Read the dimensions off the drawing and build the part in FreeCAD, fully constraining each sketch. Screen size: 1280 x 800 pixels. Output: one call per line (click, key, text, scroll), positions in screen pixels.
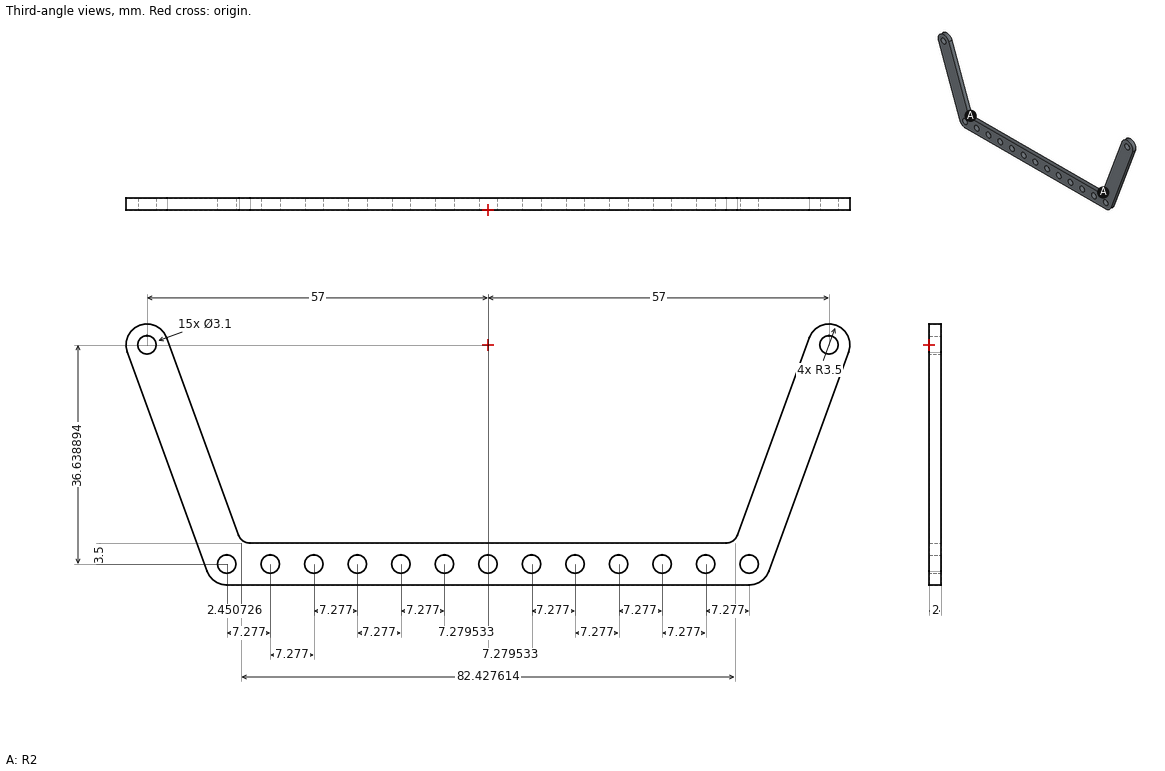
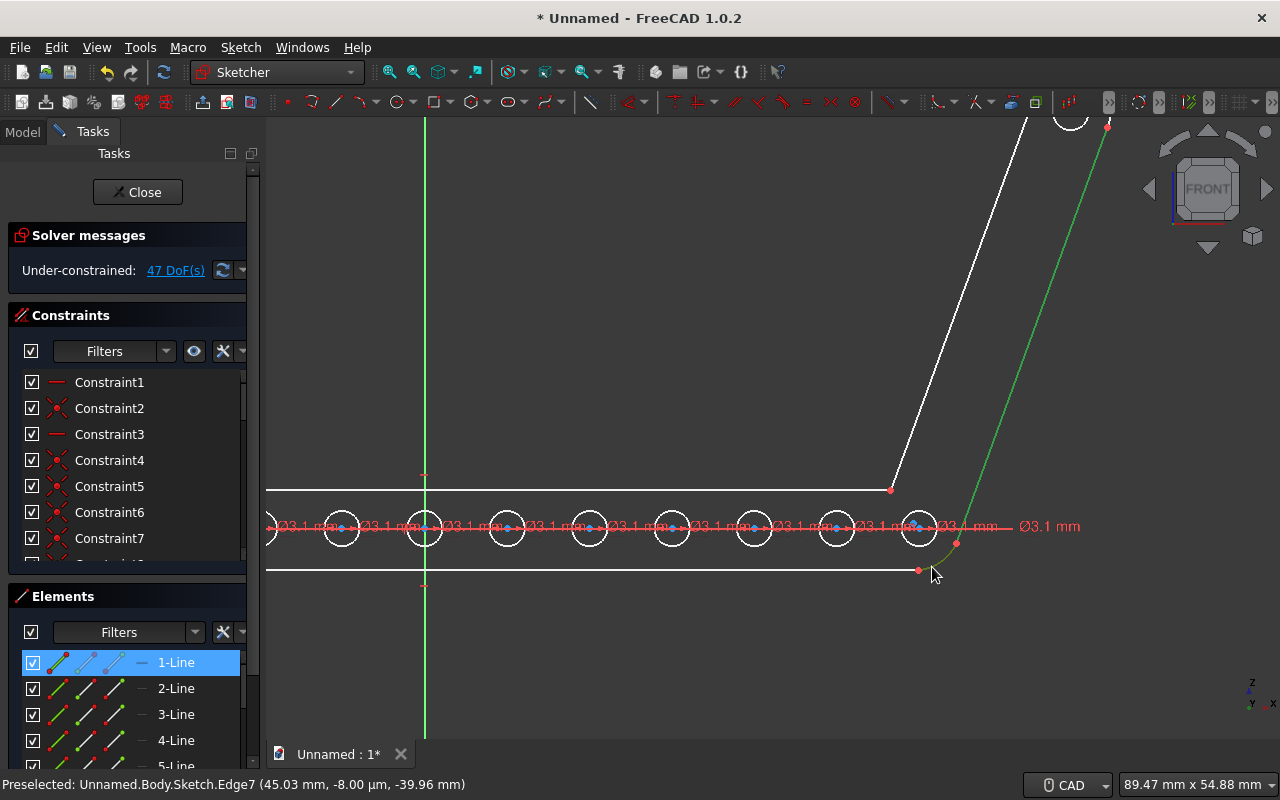
click(784, 102)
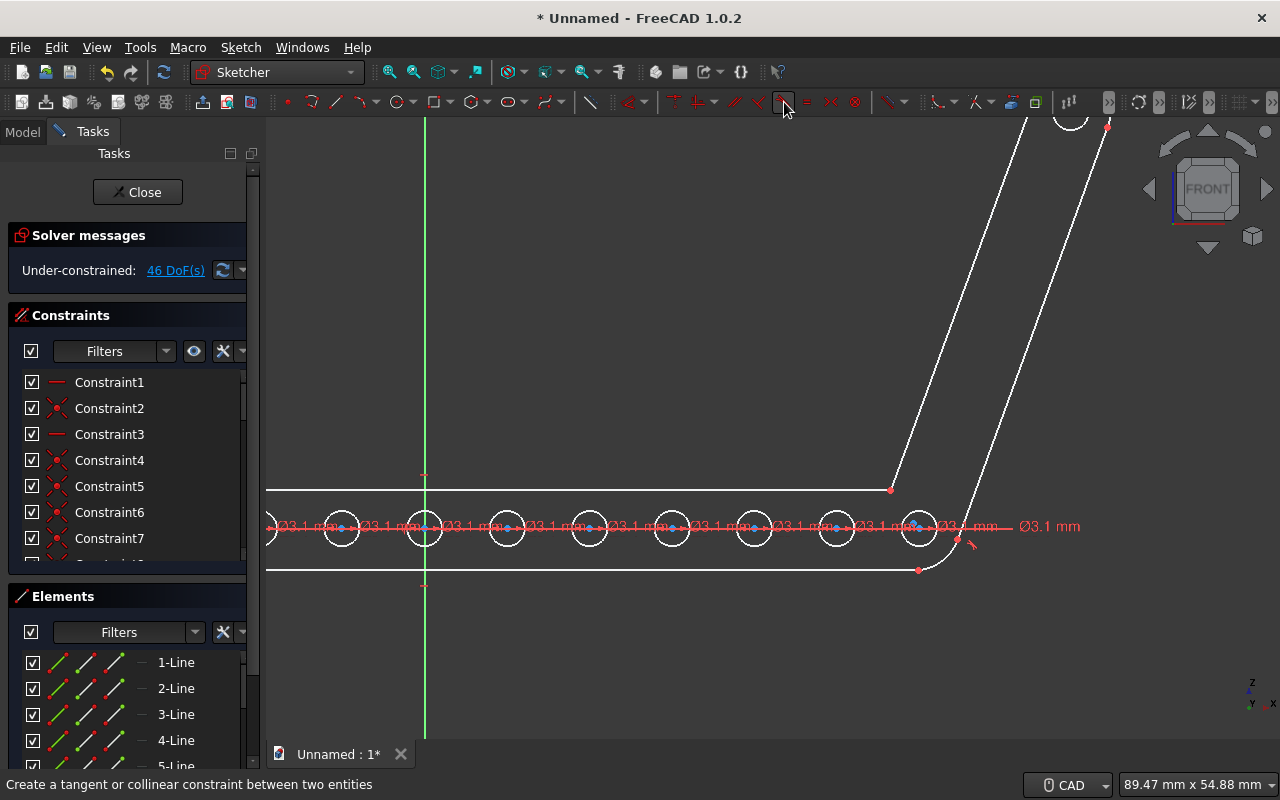
click(1063, 251)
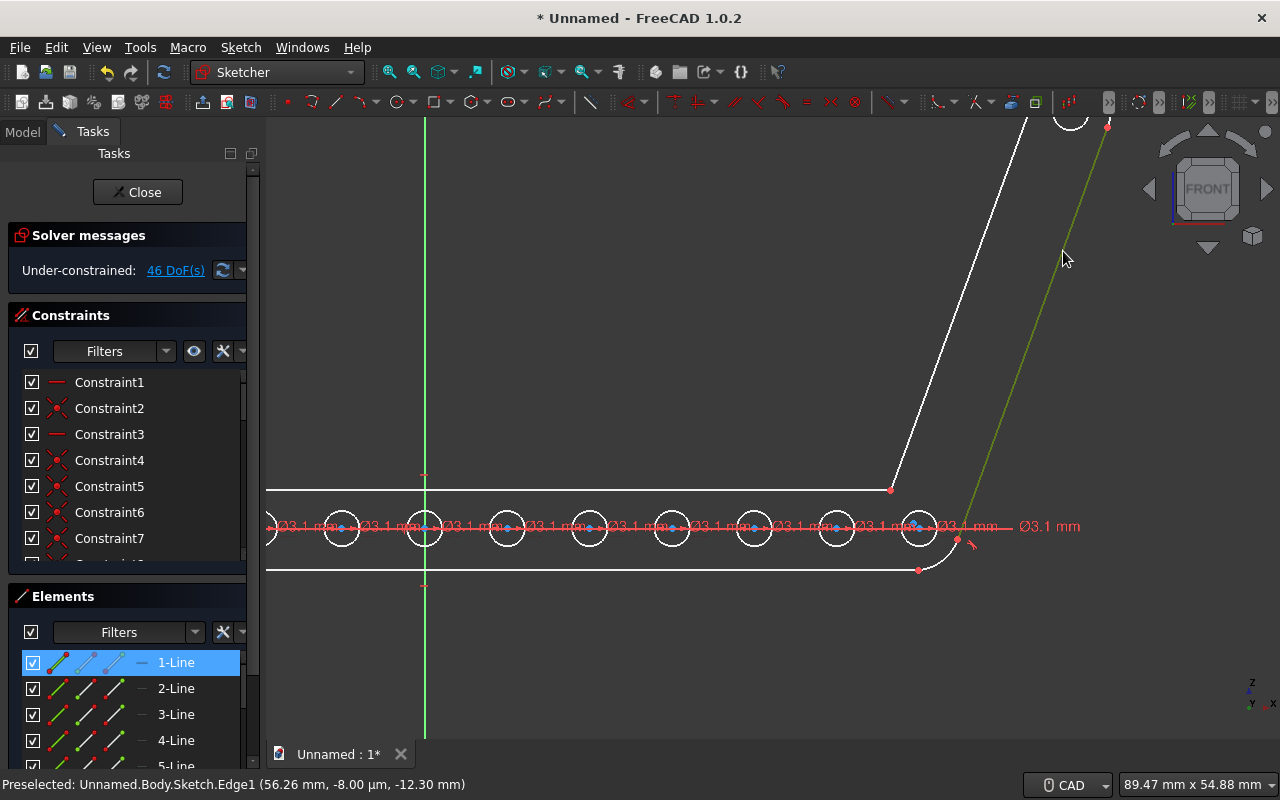
scroll(933, 515, down, 4)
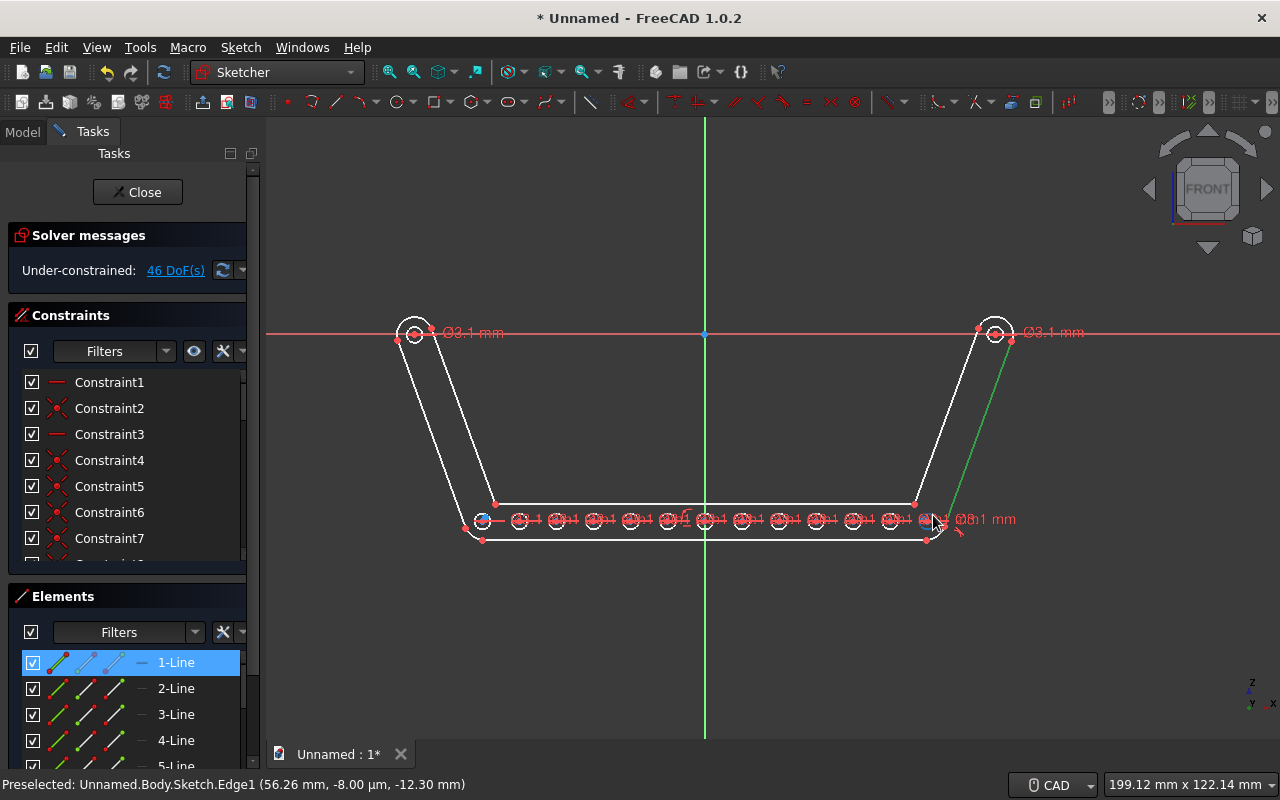
scroll(1010, 325, up, 2)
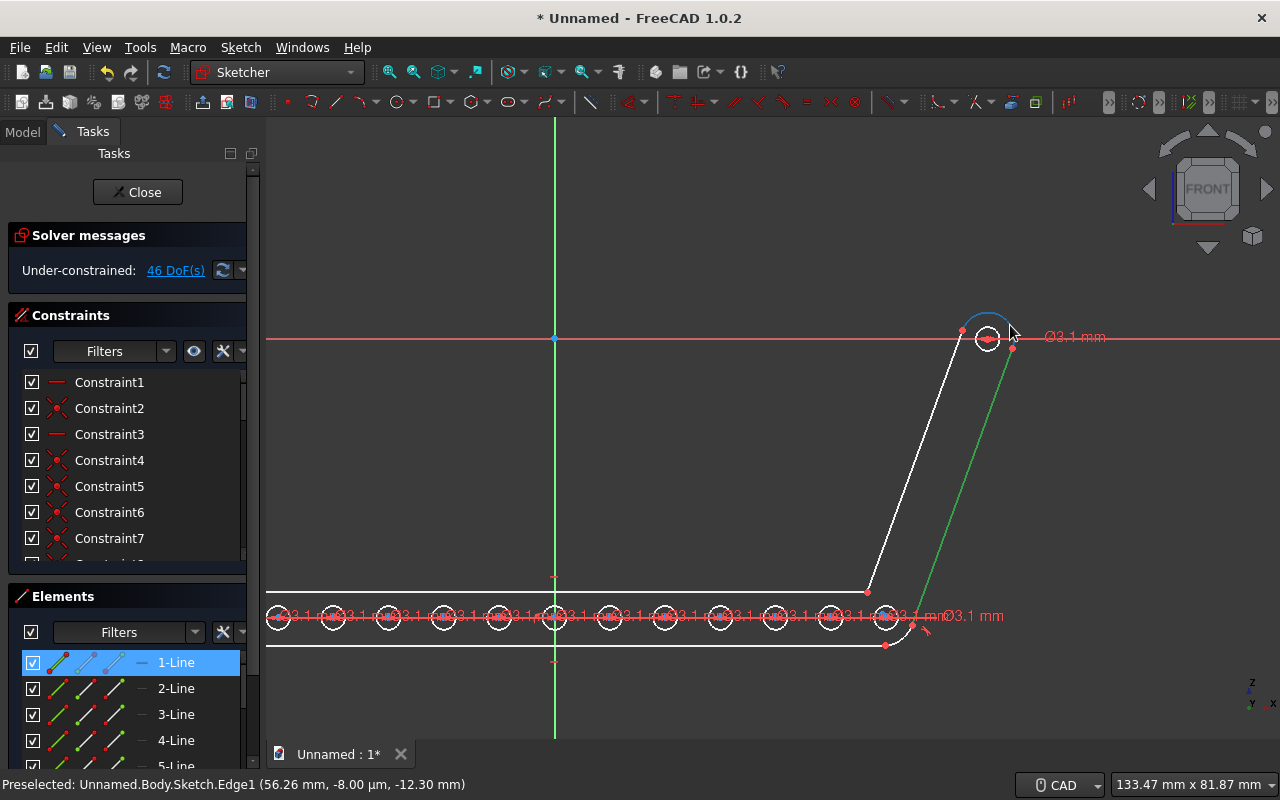
click(1010, 325)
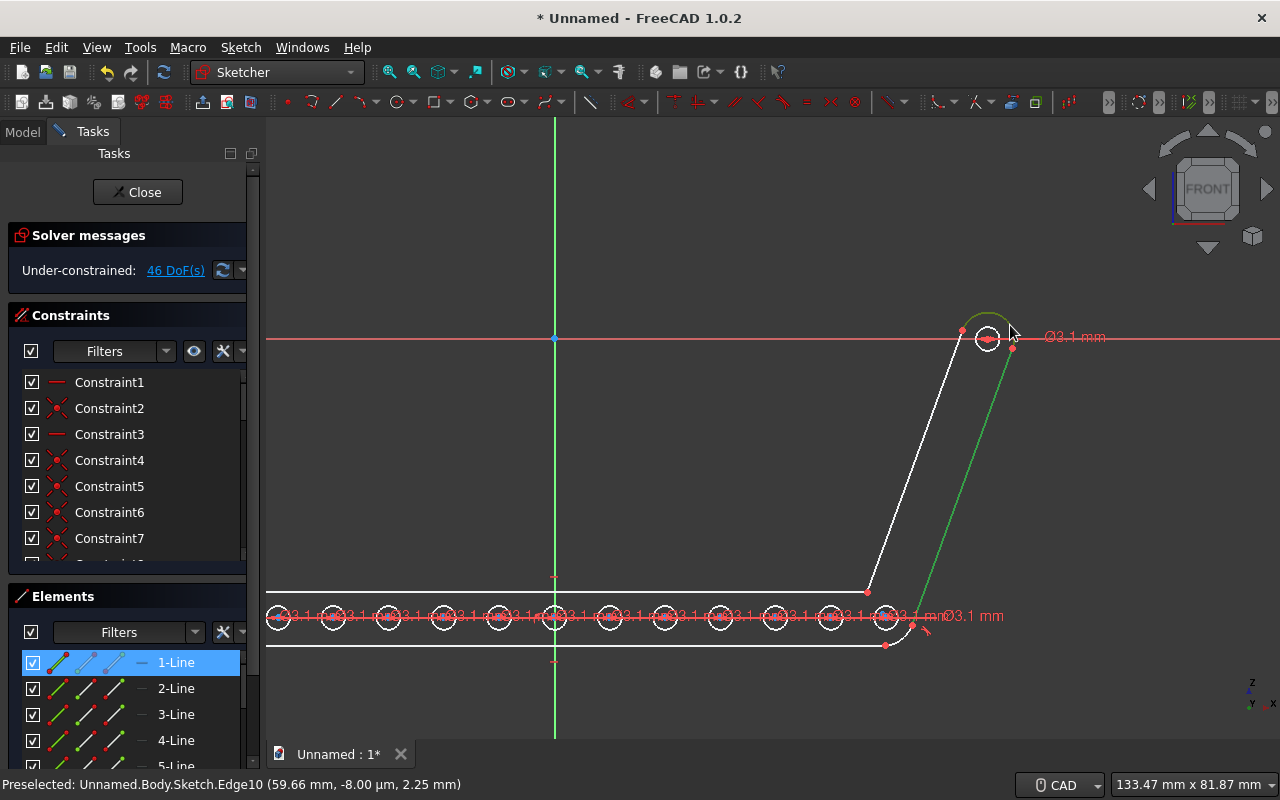
key(t)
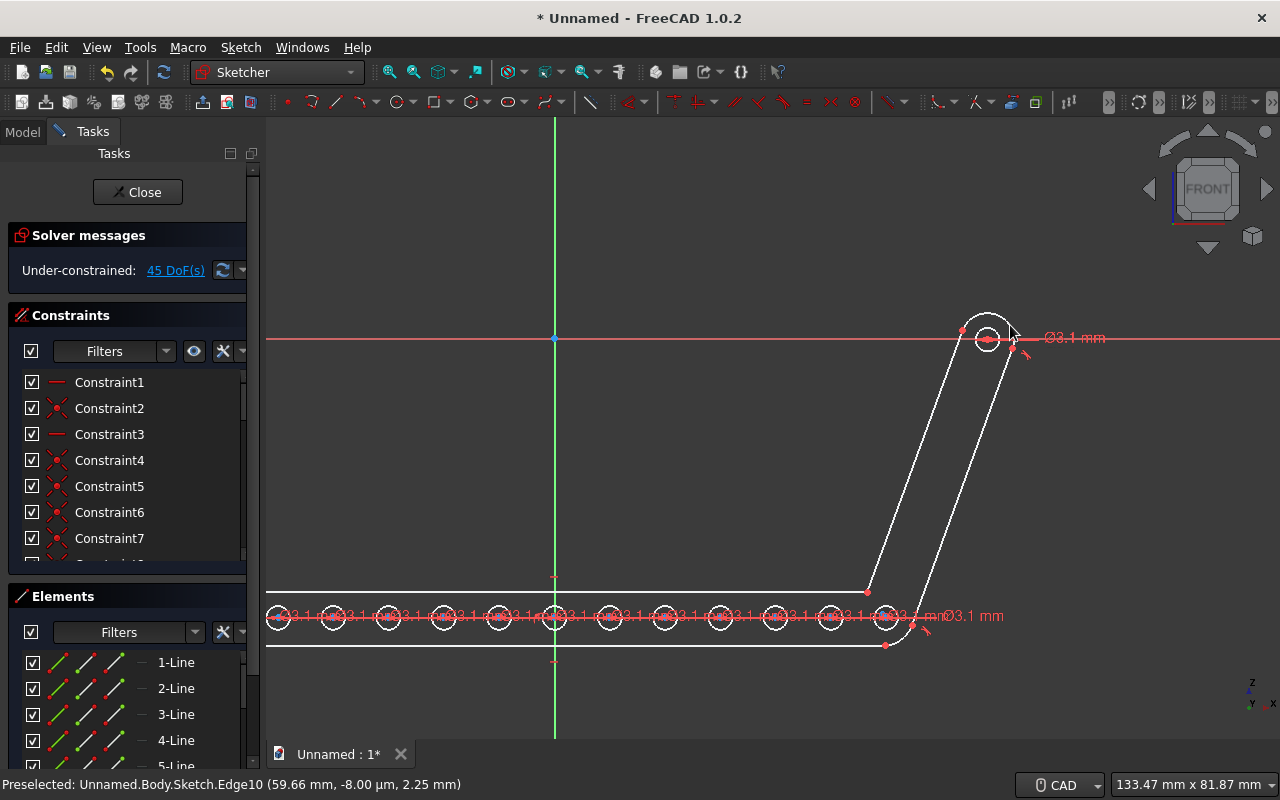
click(687, 646)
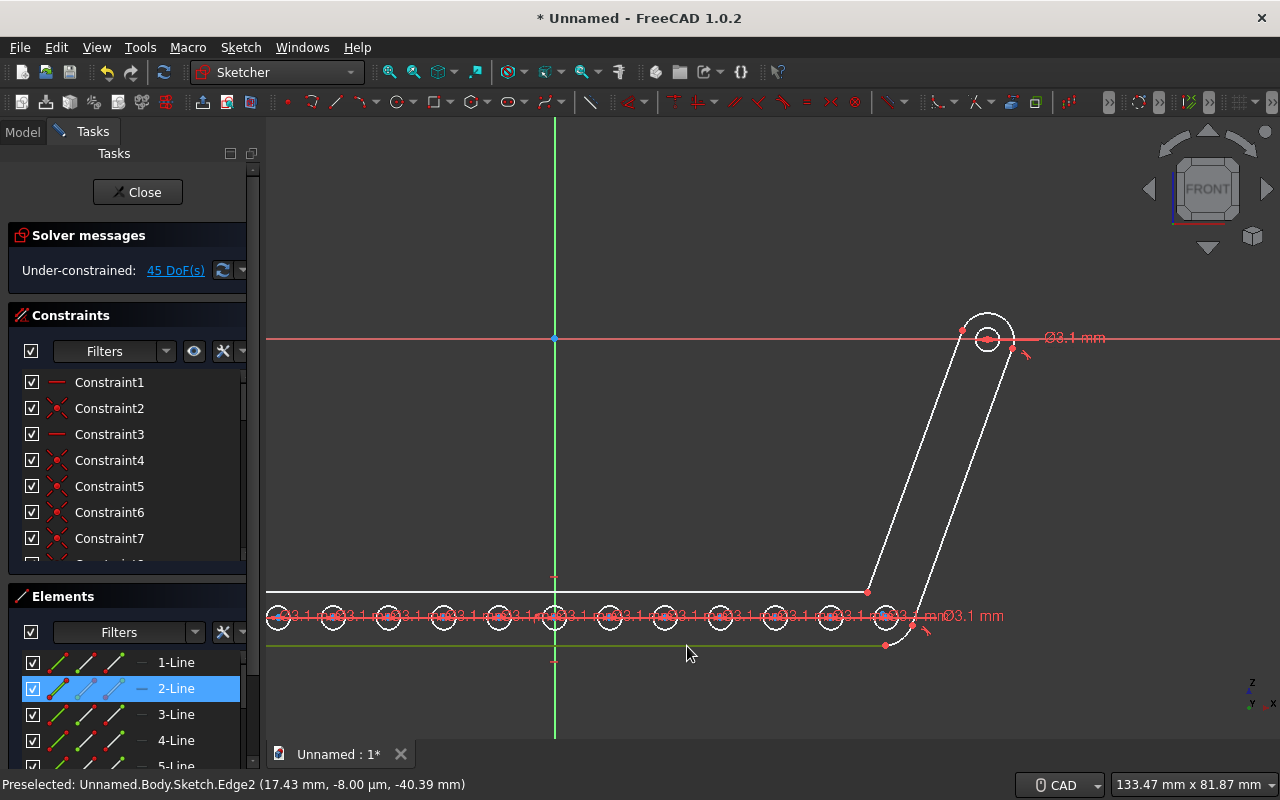
scroll(896, 643, up, 2)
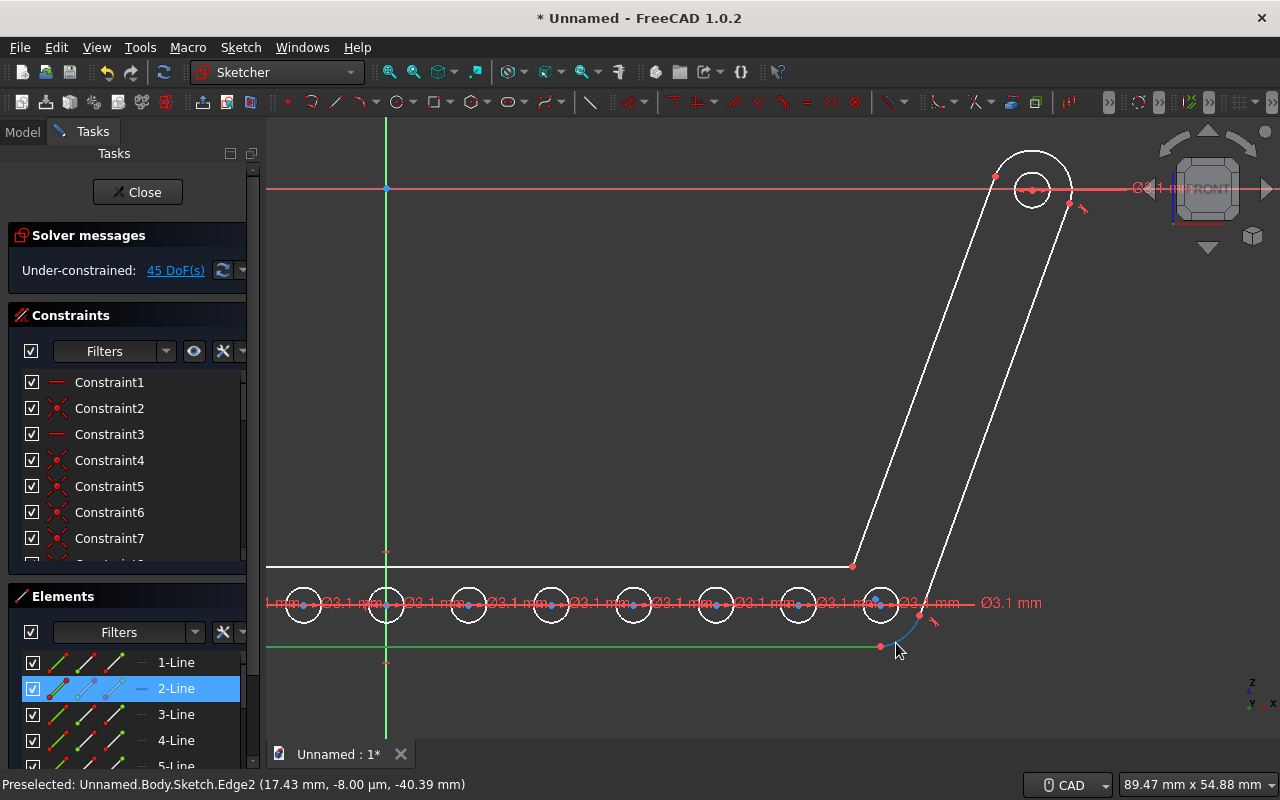
click(895, 643)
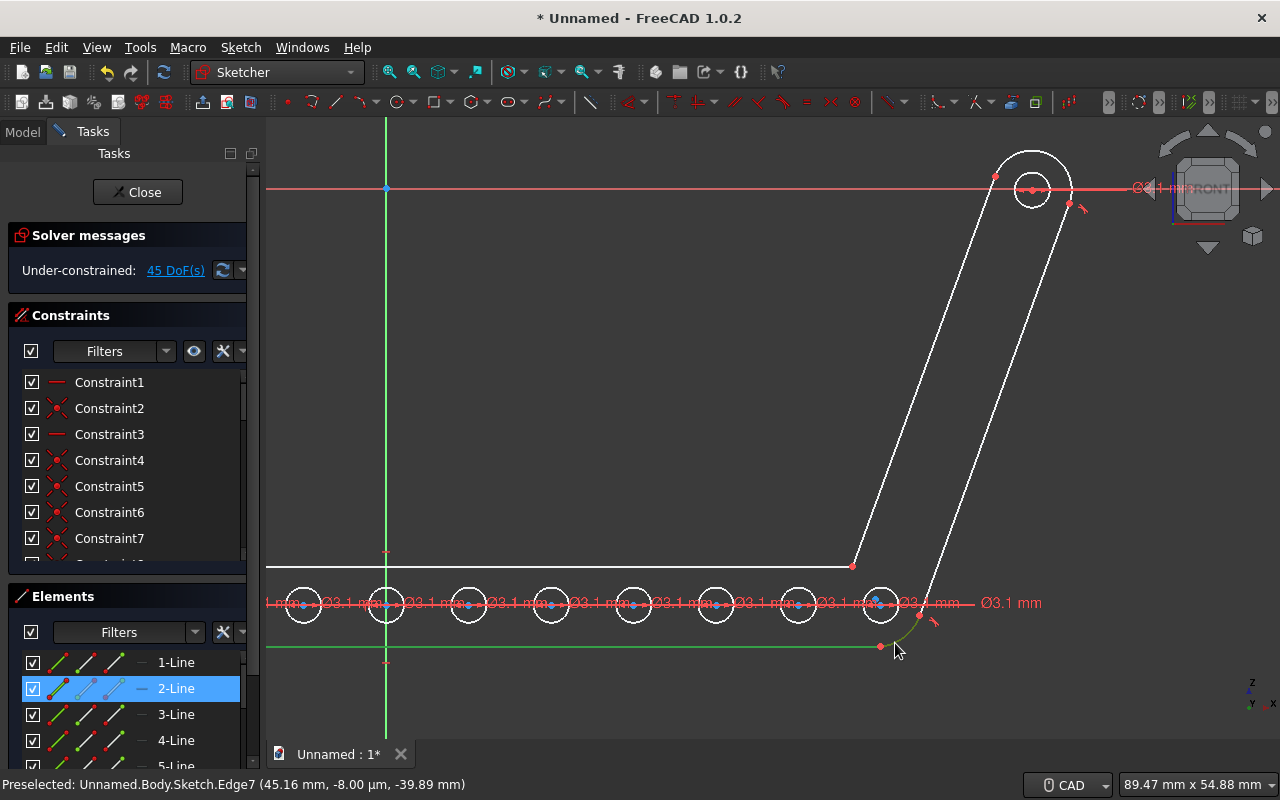
key(t)